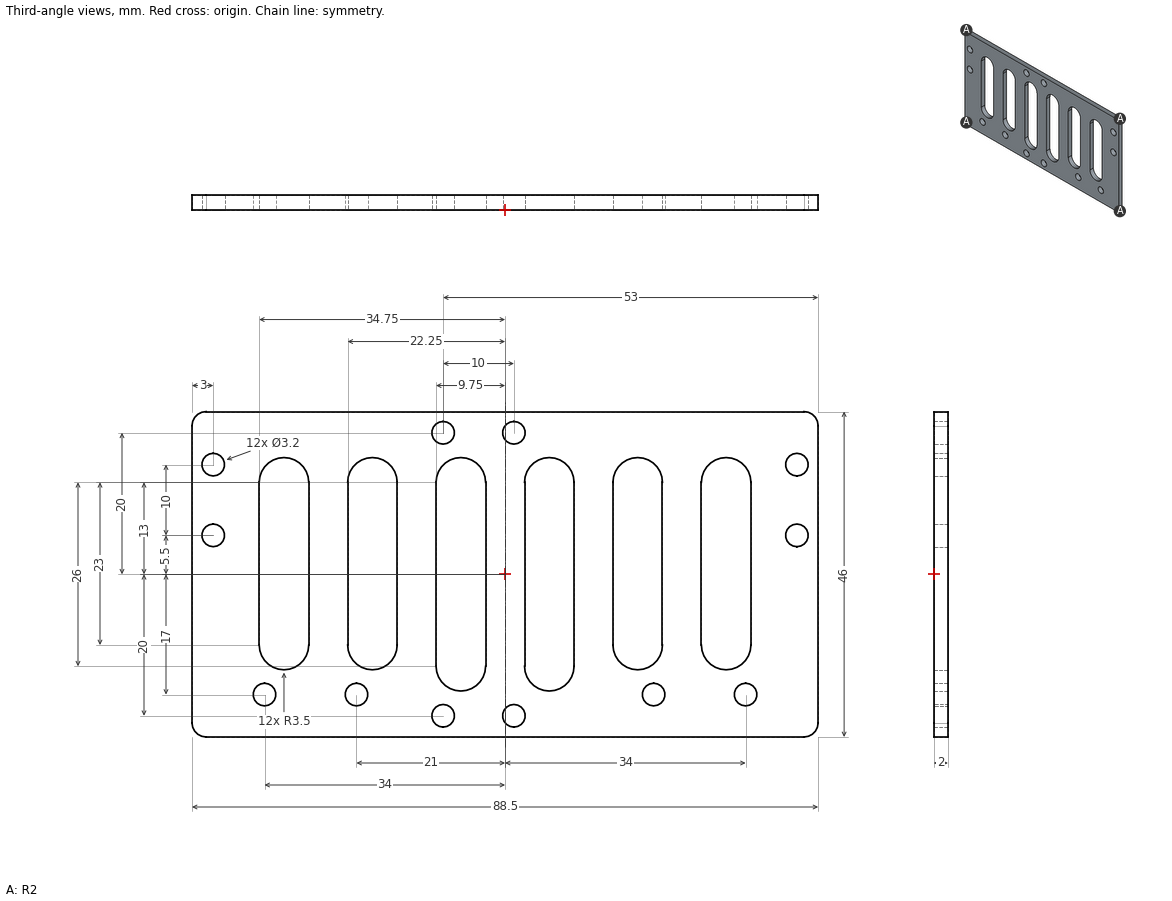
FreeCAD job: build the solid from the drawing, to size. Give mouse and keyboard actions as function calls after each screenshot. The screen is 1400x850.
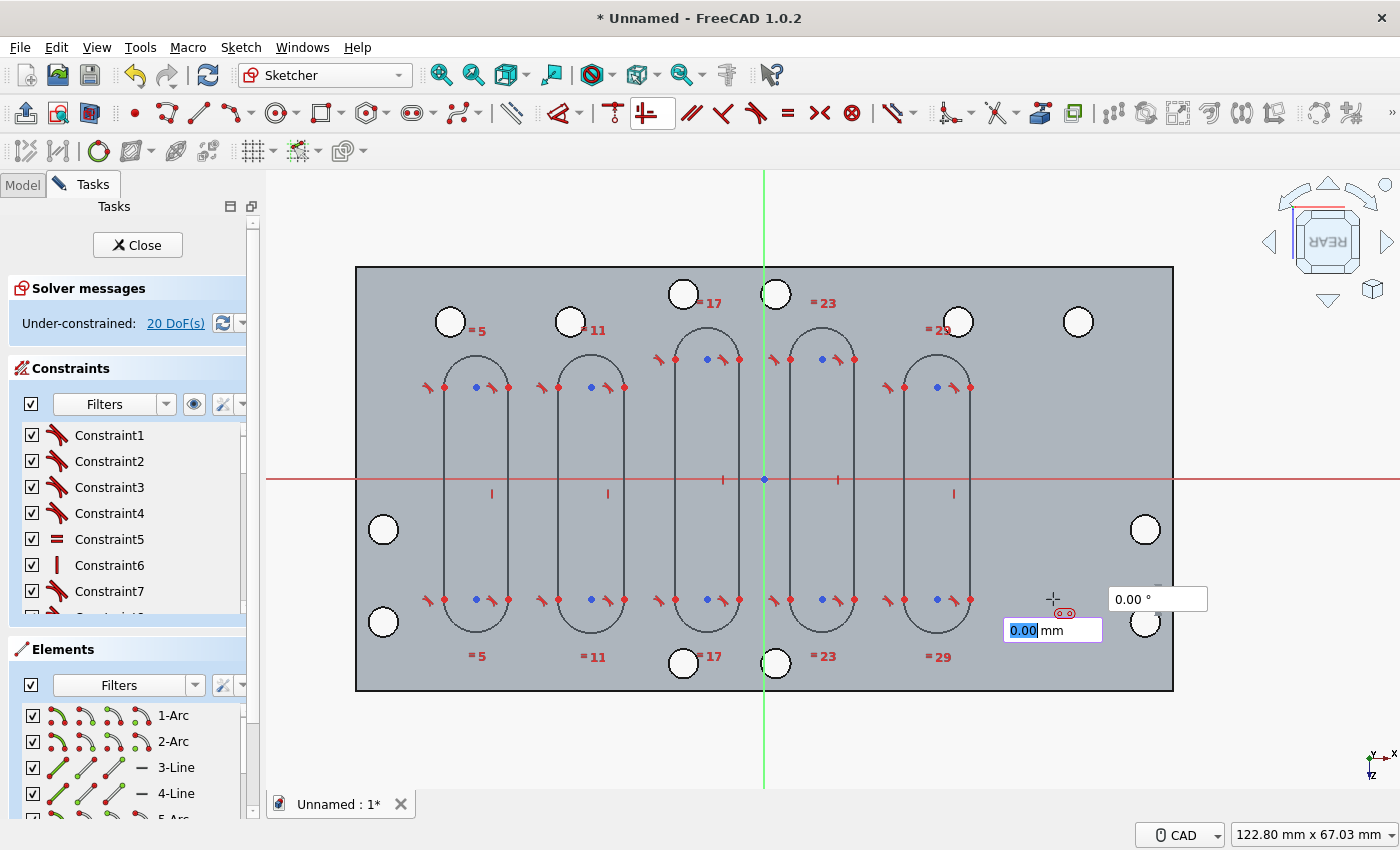
click(1053, 387)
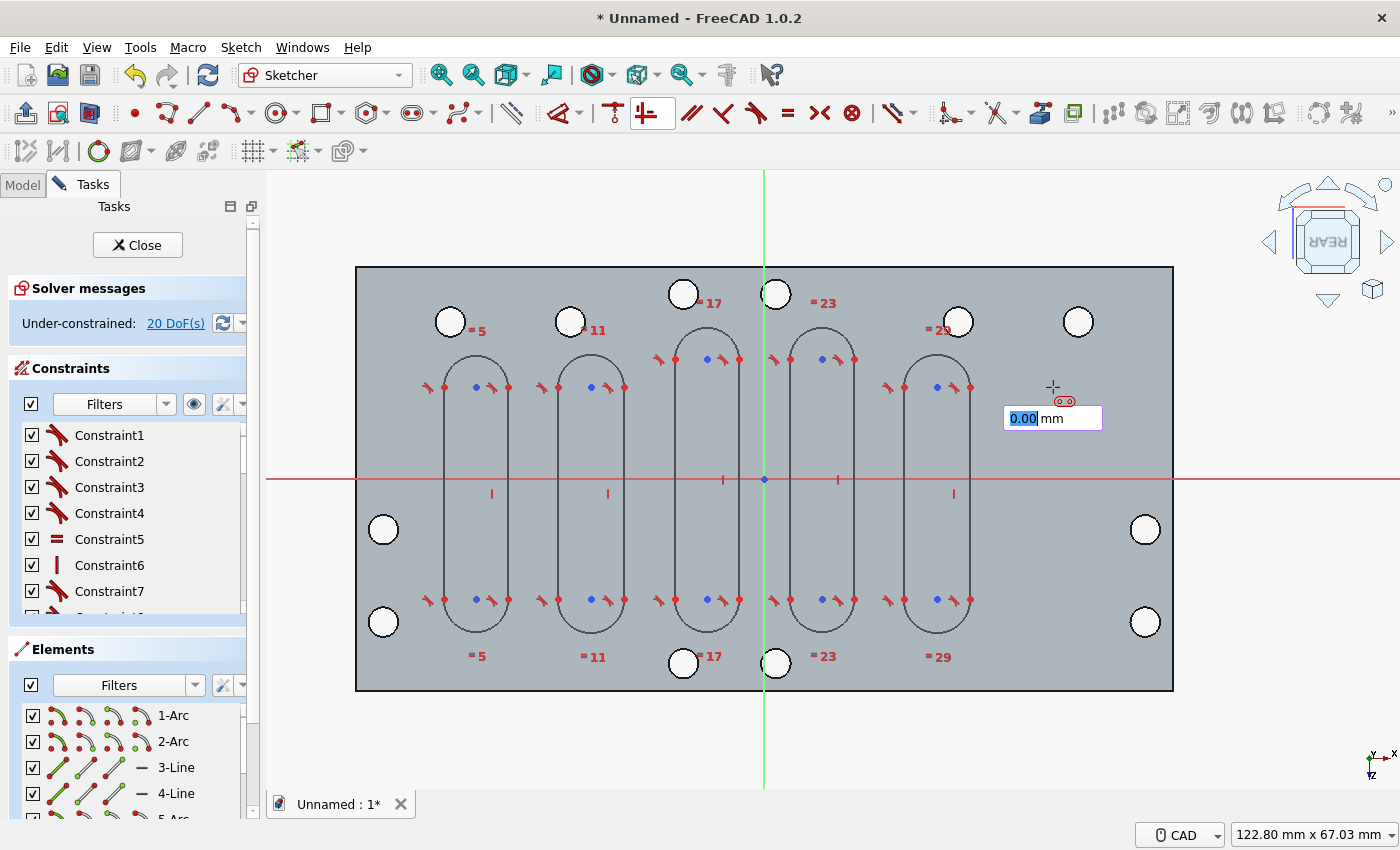
click(1085, 525)
key(Escape)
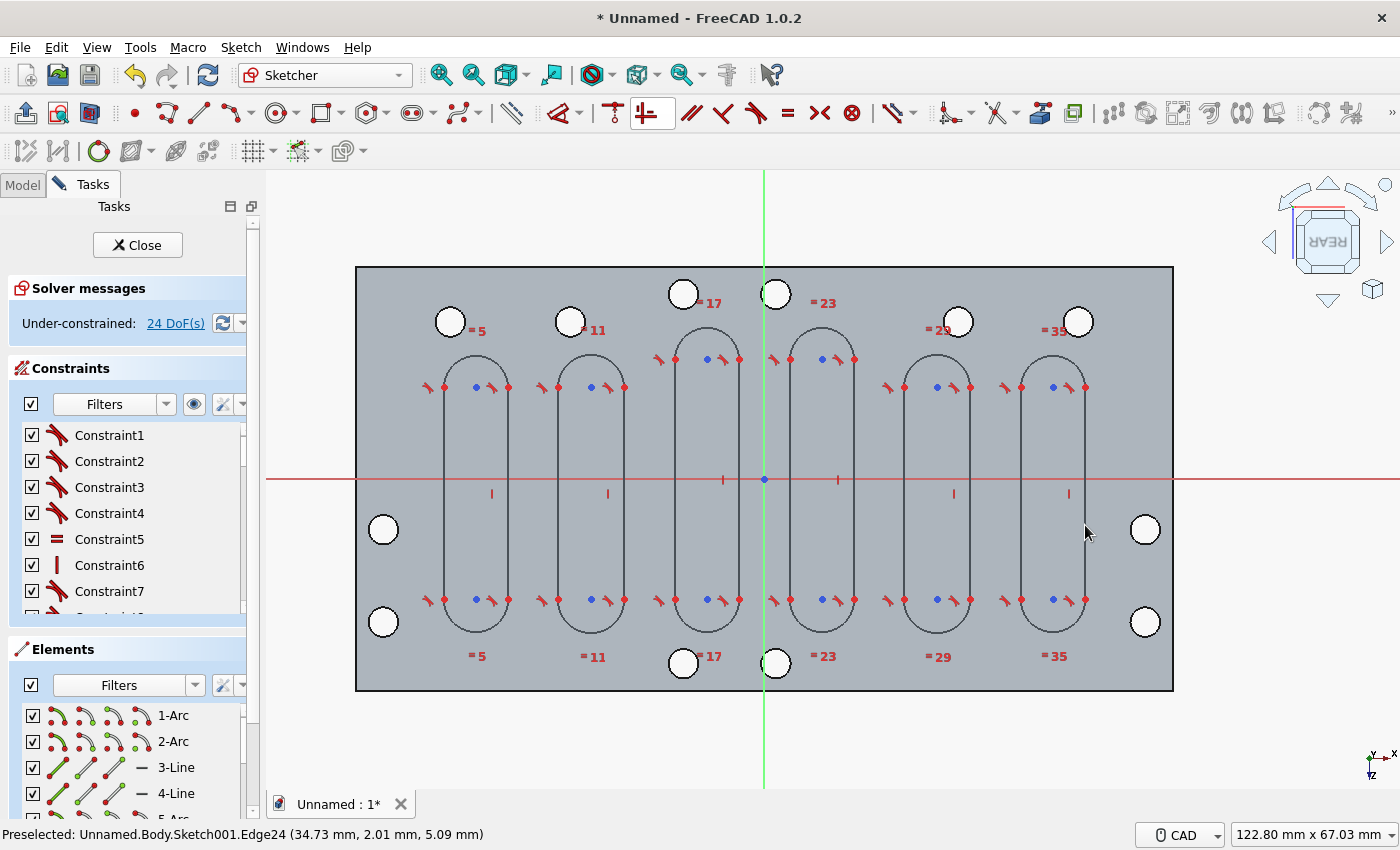
click(457, 626)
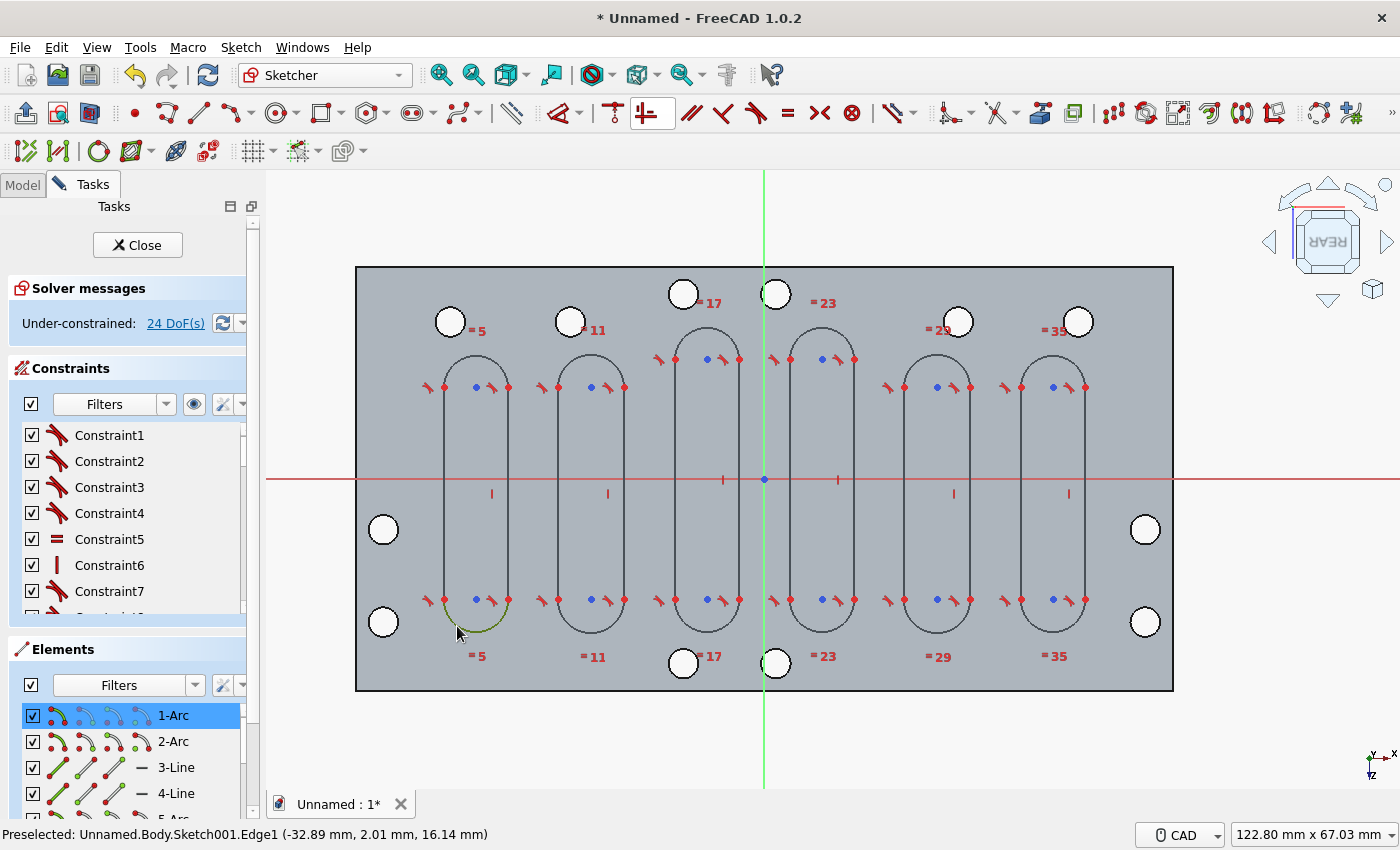
click(572, 627)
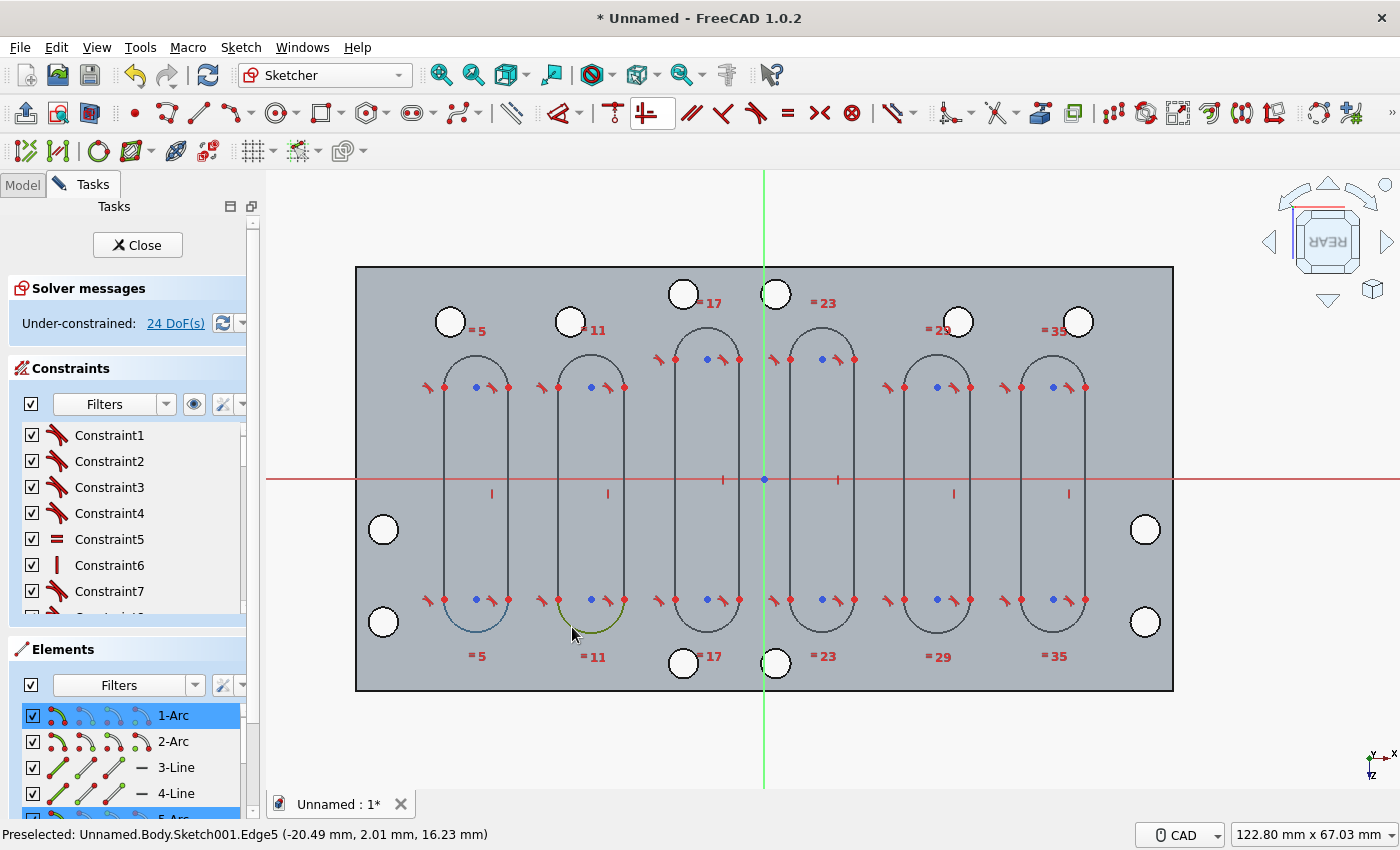
click(688, 626)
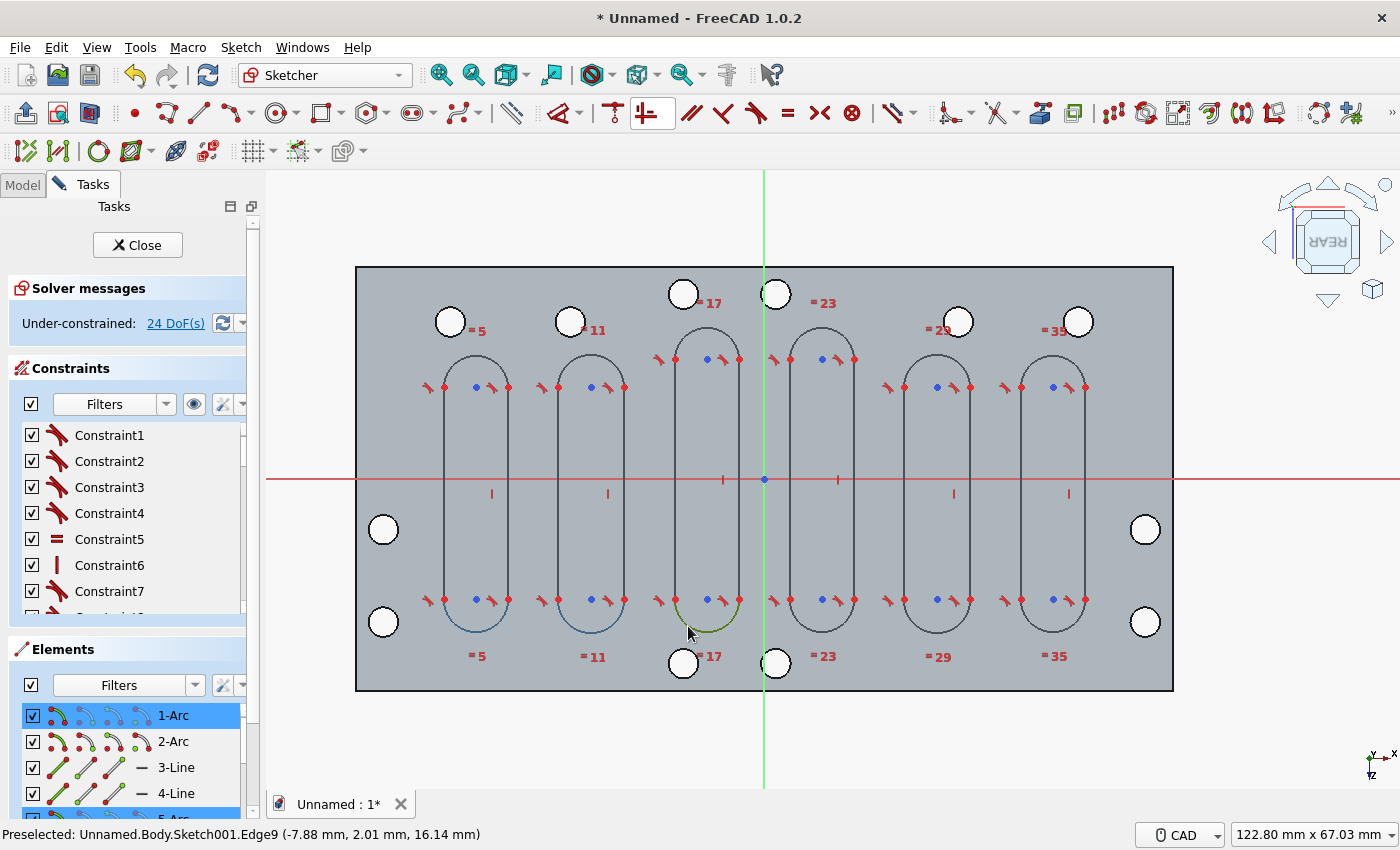
click(803, 626)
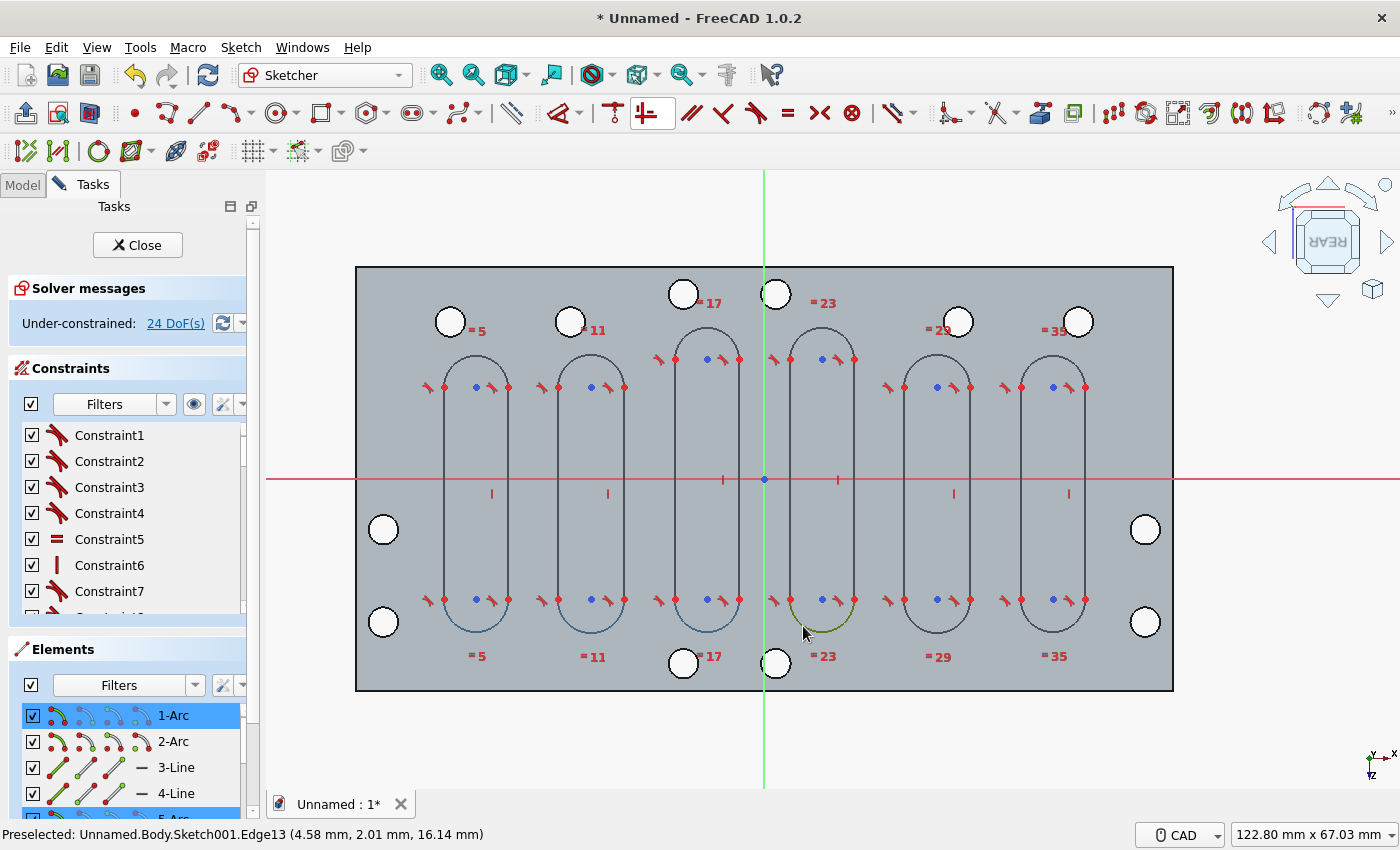
click(918, 627)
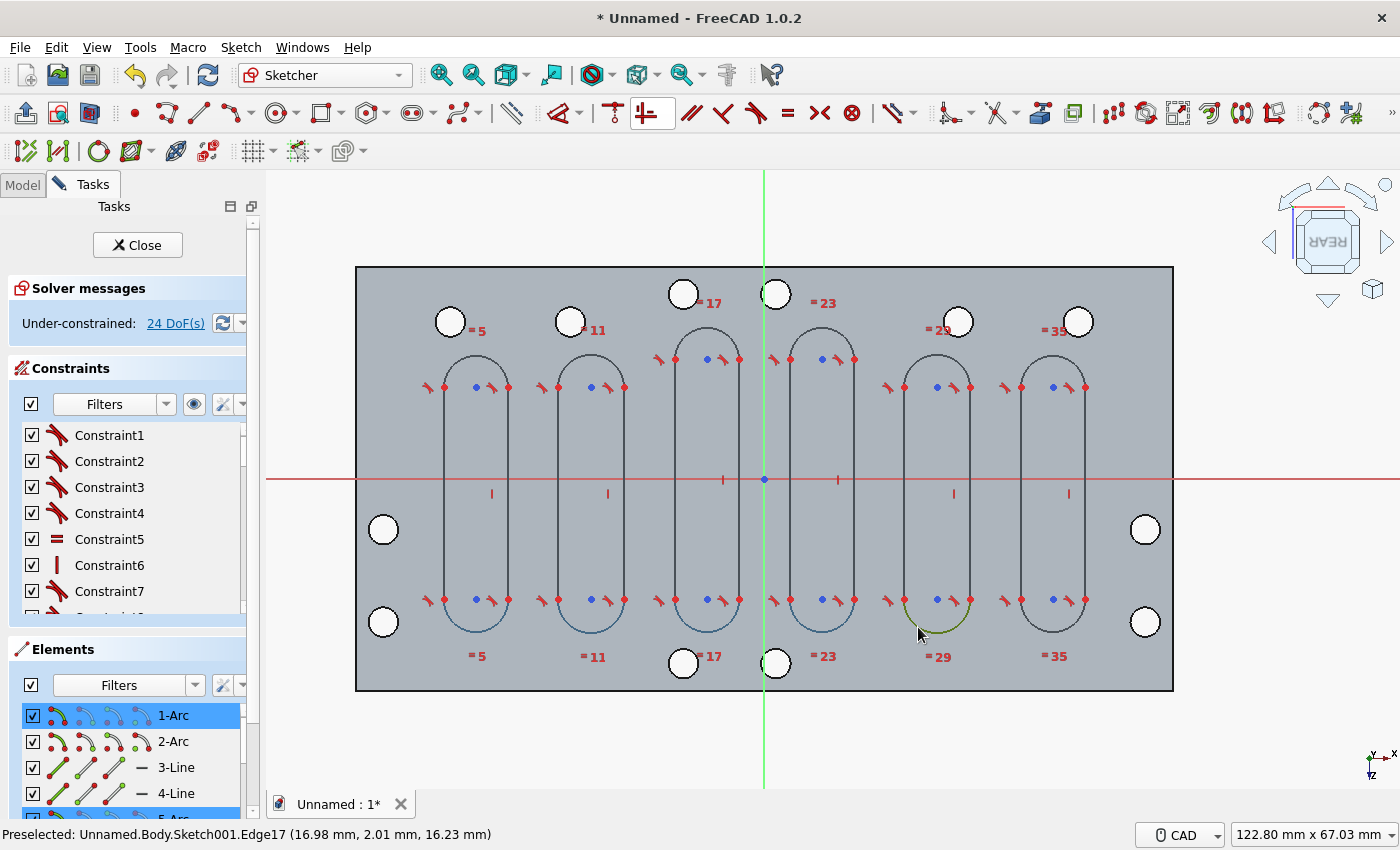
click(1034, 626)